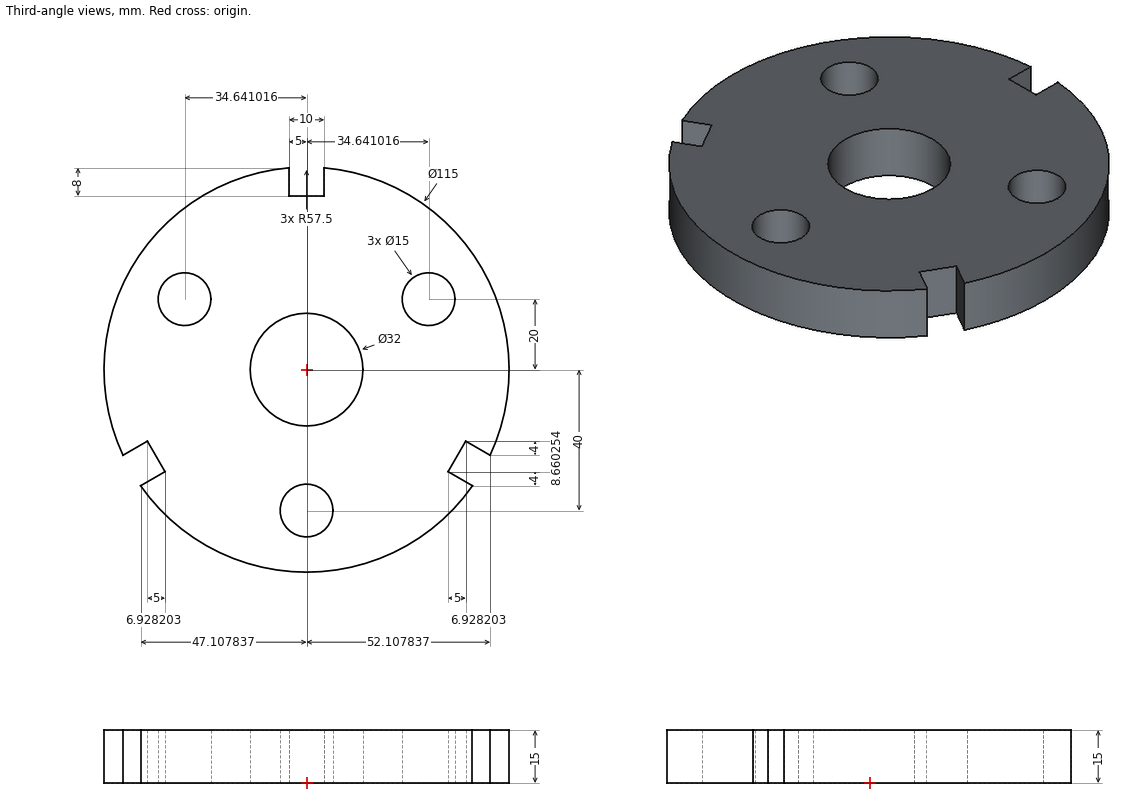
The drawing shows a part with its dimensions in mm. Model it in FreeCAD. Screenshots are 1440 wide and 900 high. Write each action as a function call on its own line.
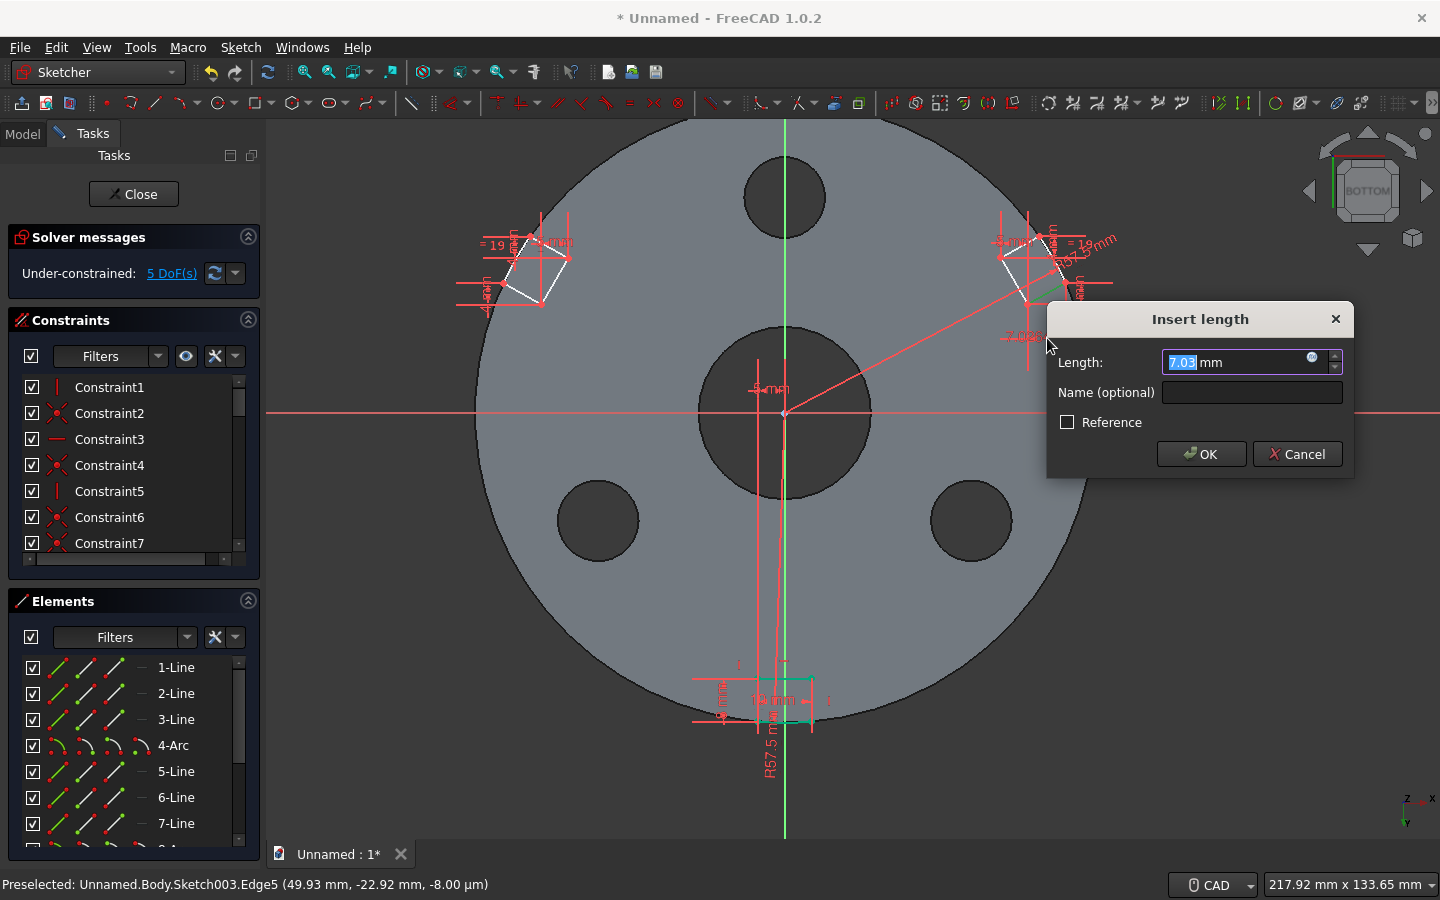
text(6.928203)
key(Return)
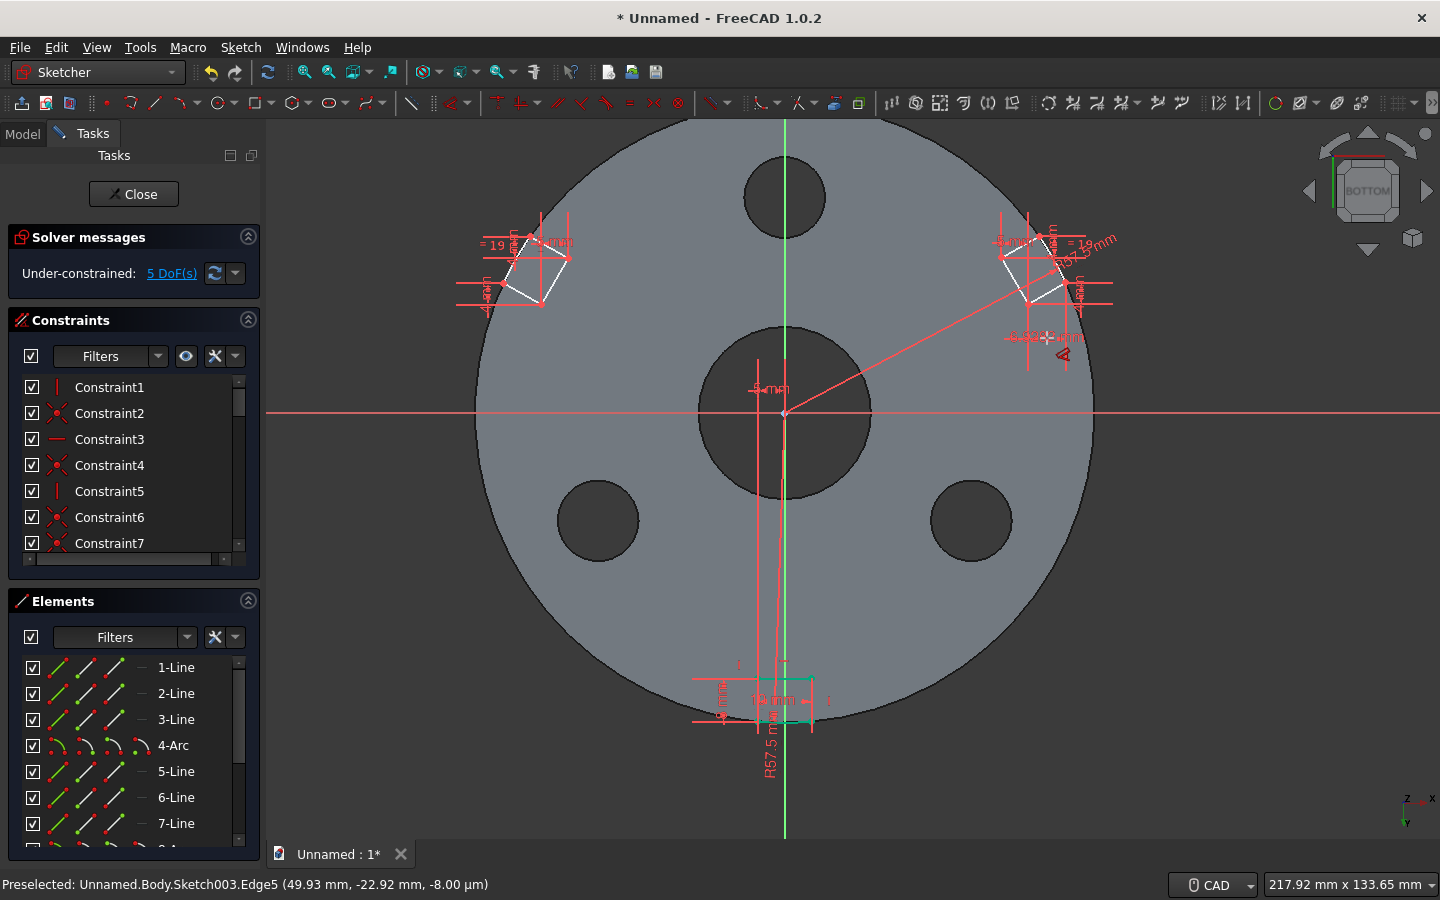
click(1020, 290)
click(967, 281)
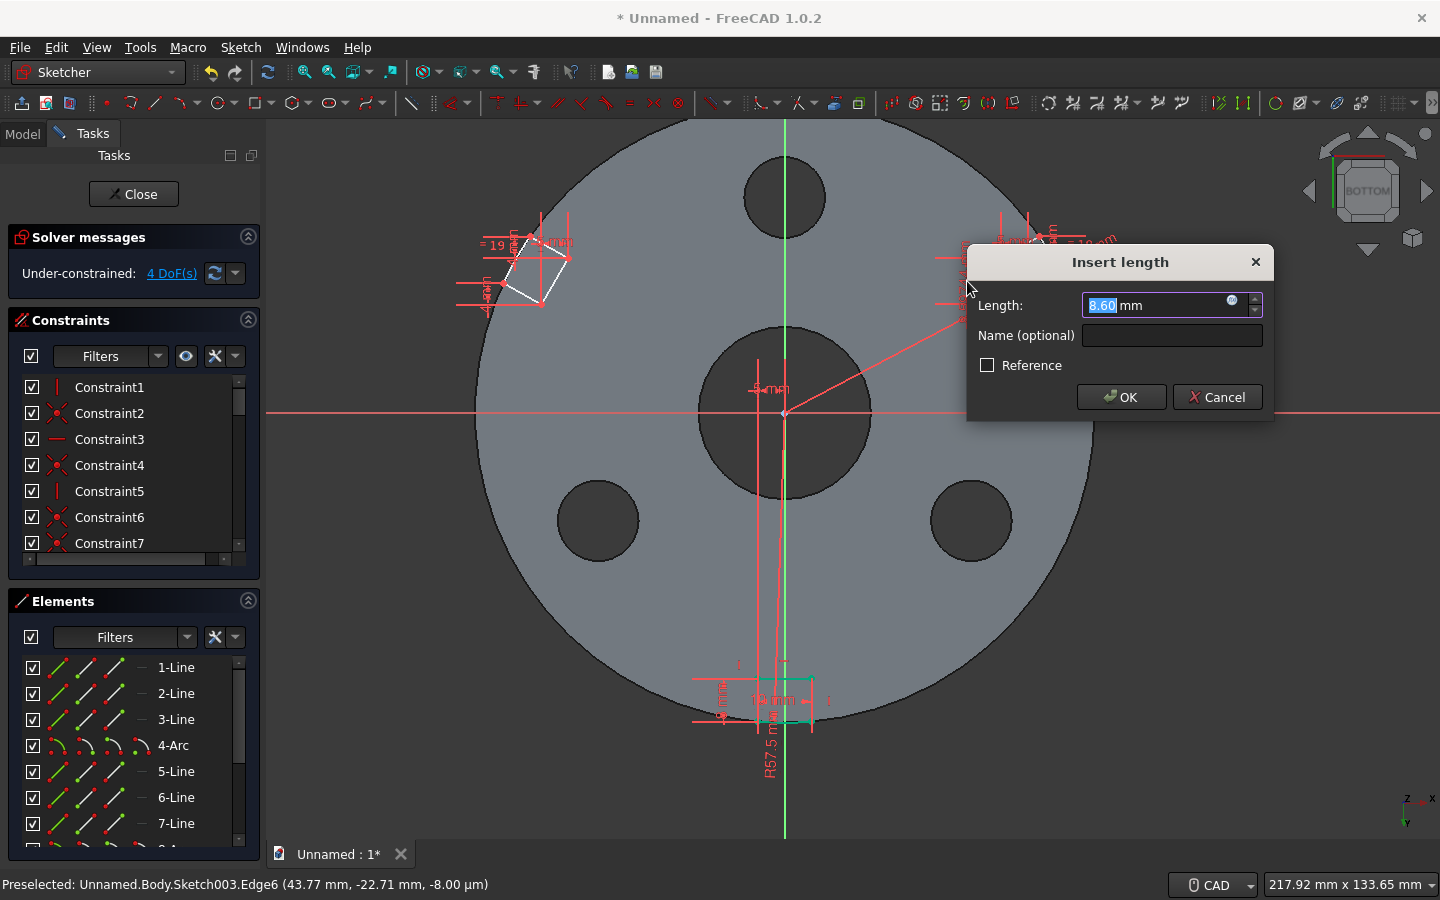
text(8.660254)
key(Return)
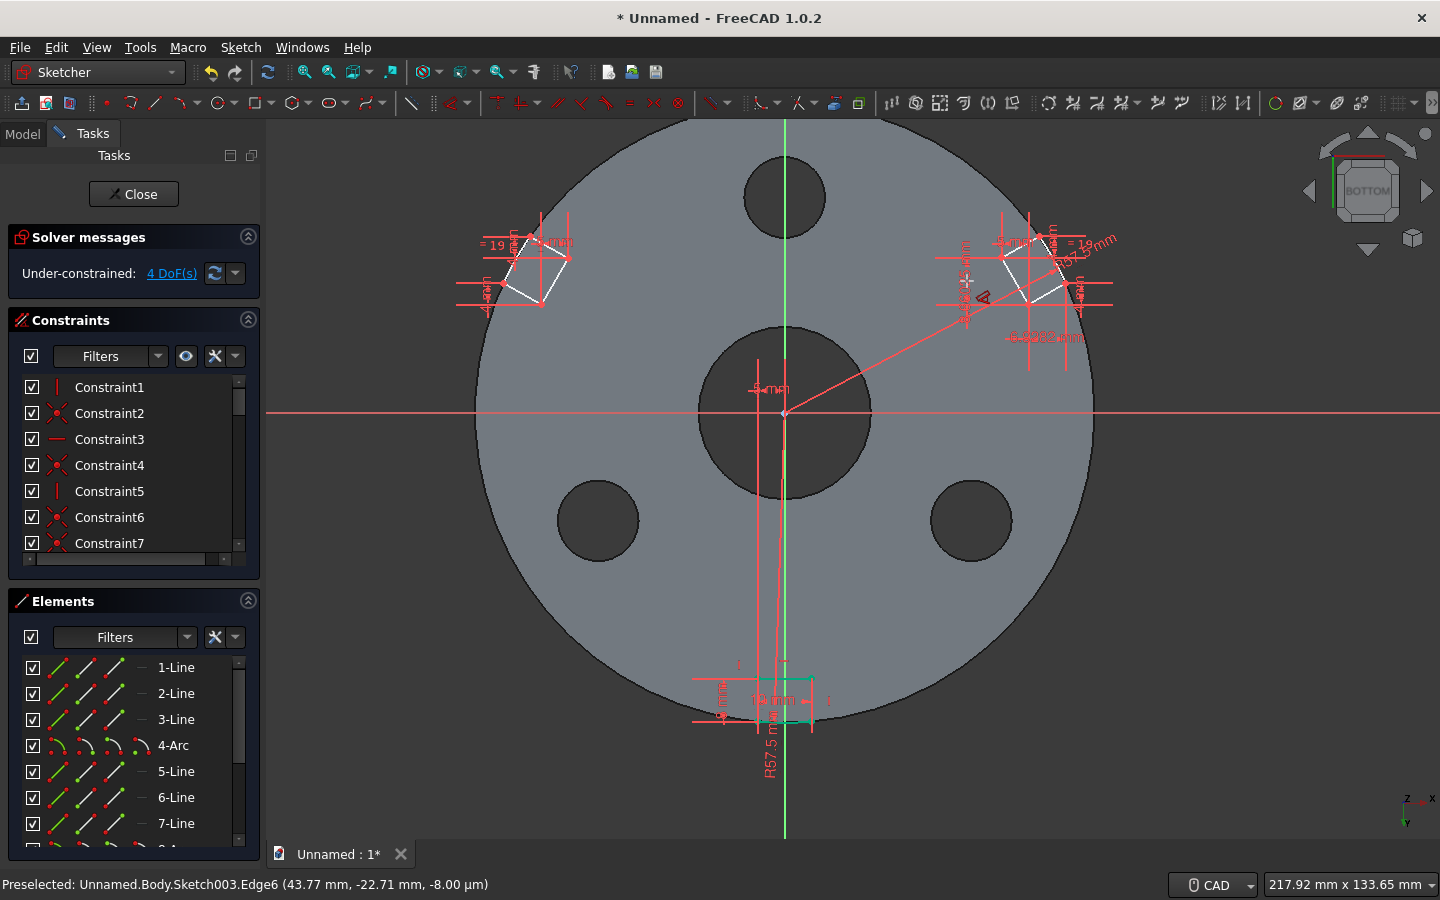
click(542, 243)
click(549, 203)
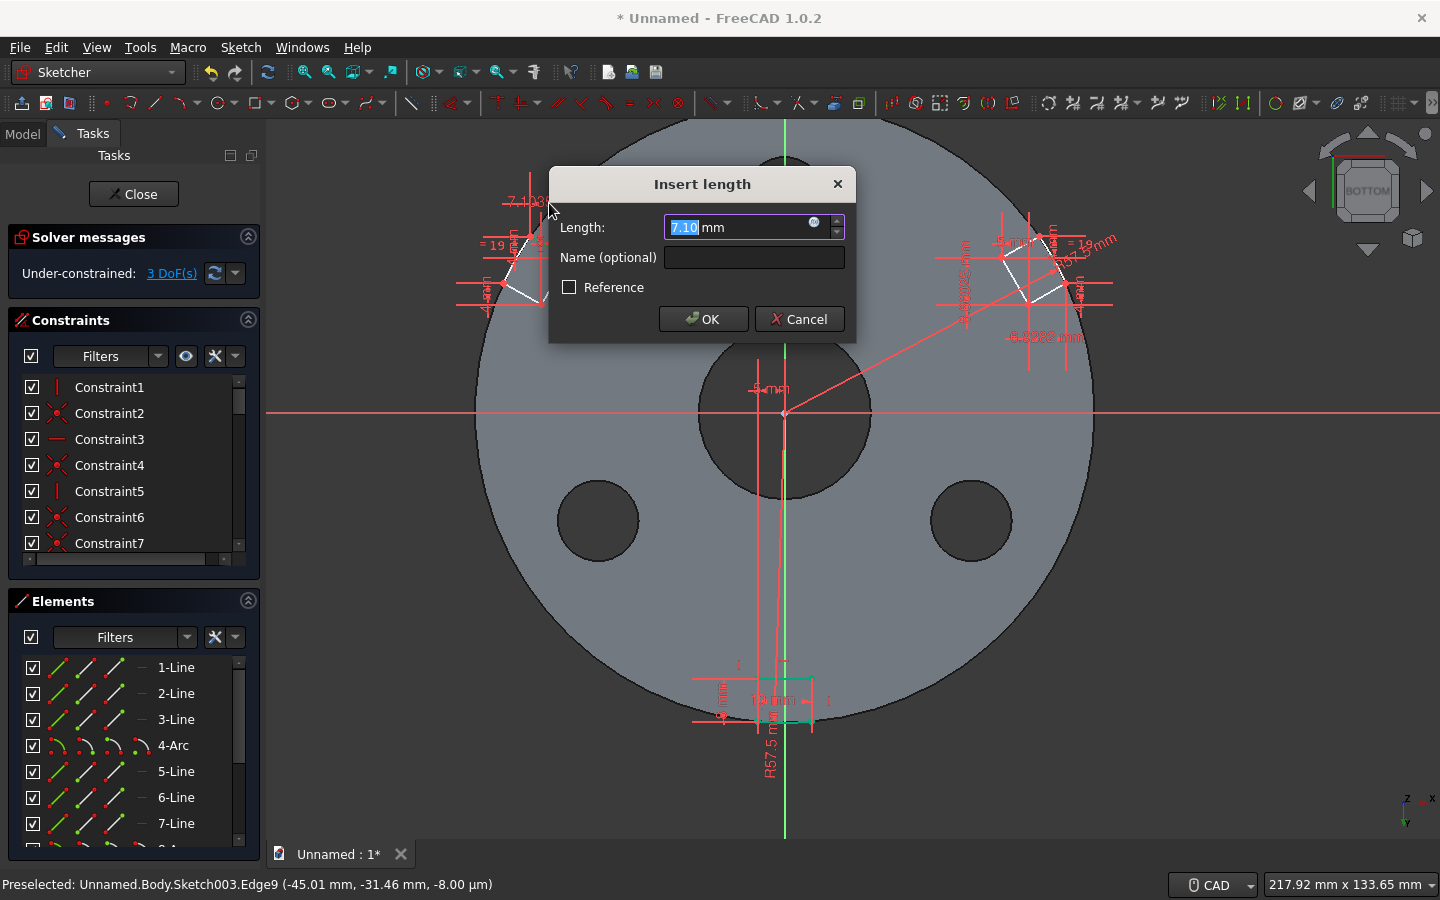
text(6.928203)
key(Return)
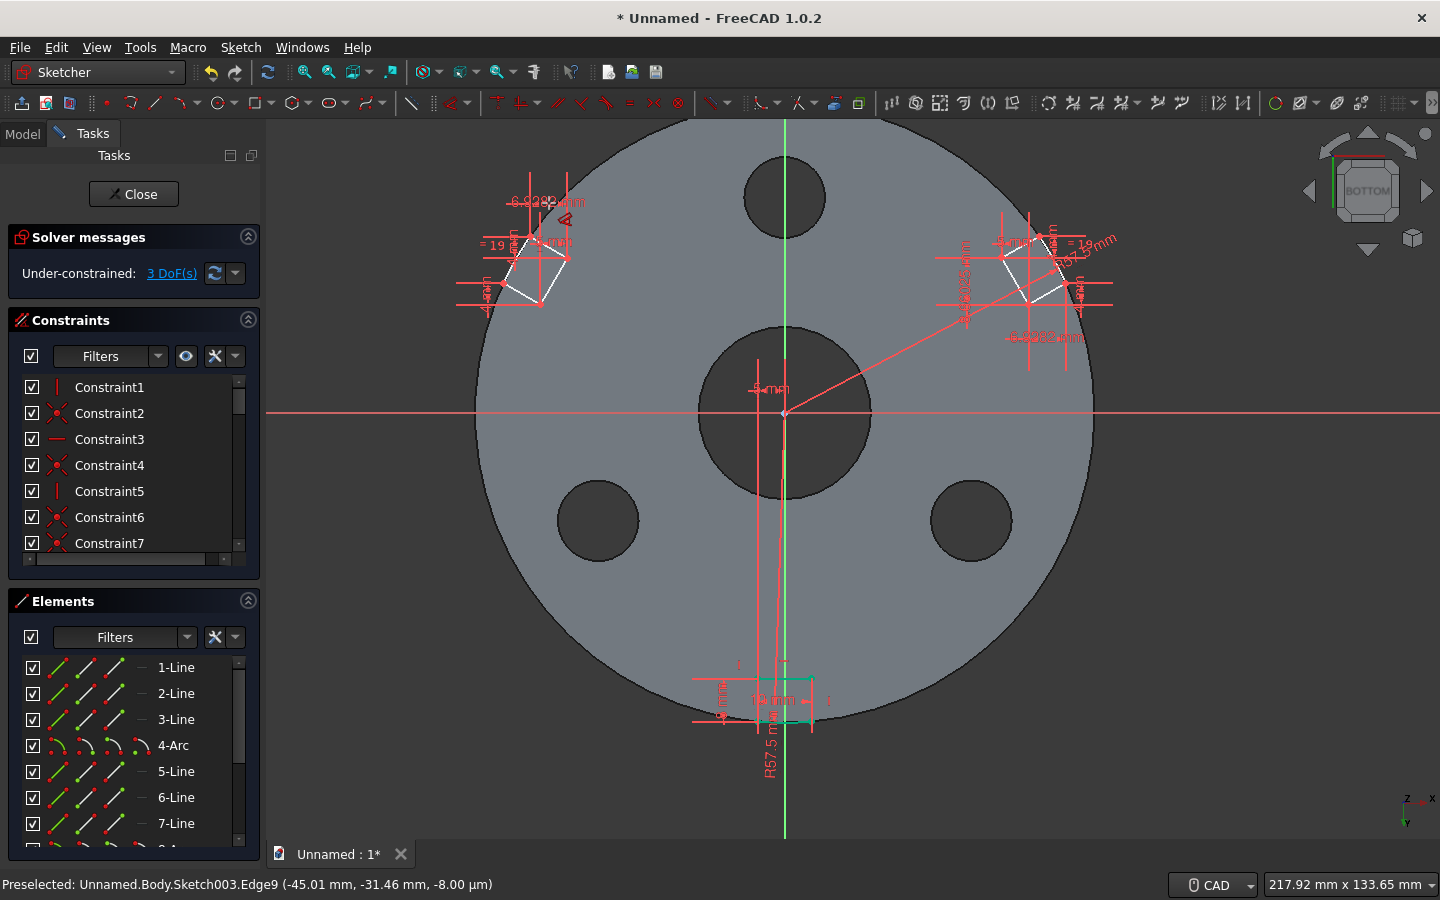
click(559, 272)
click(601, 281)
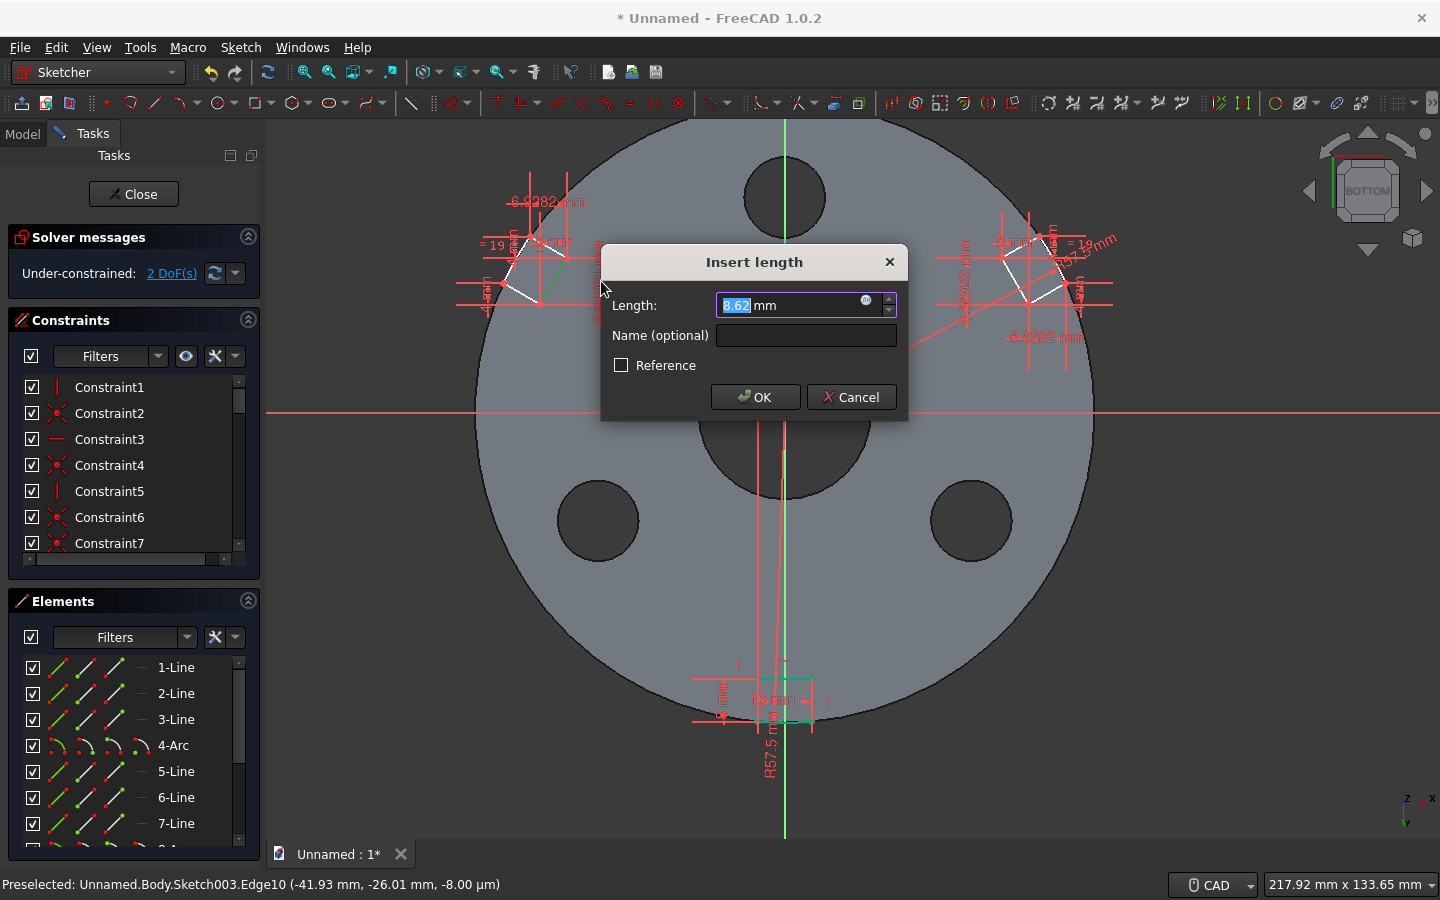
text(8.660254)
key(Return)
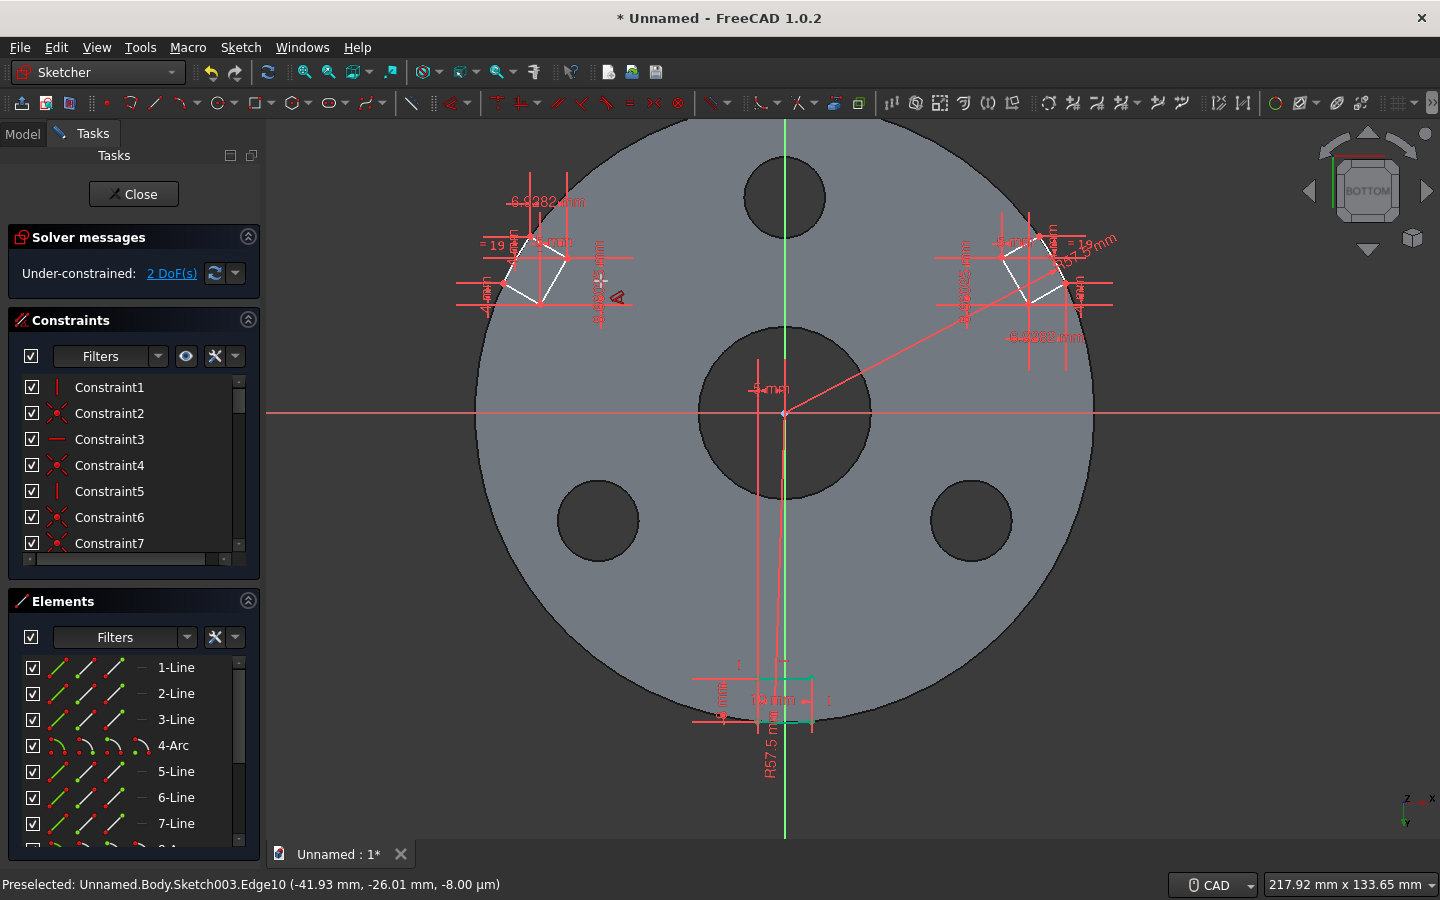
click(1066, 283)
click(925, 249)